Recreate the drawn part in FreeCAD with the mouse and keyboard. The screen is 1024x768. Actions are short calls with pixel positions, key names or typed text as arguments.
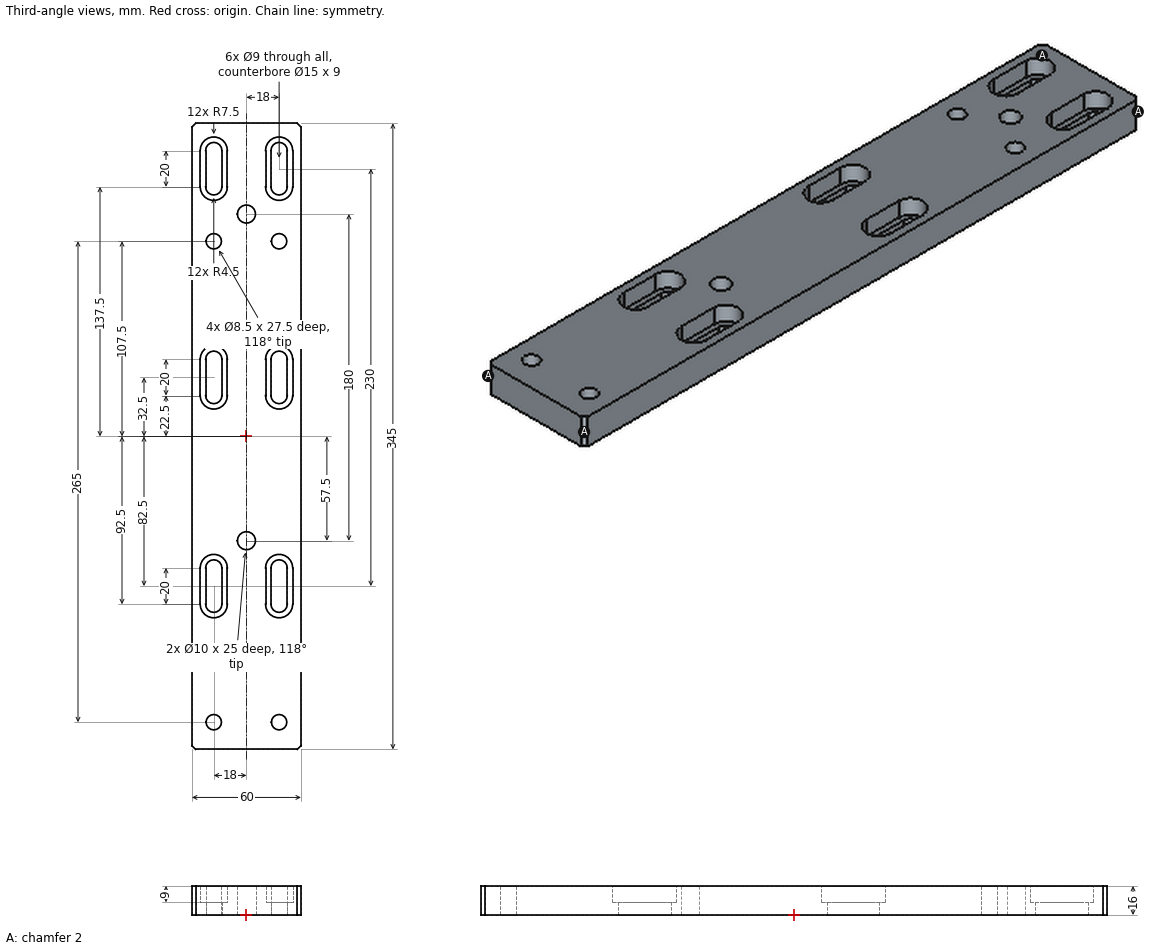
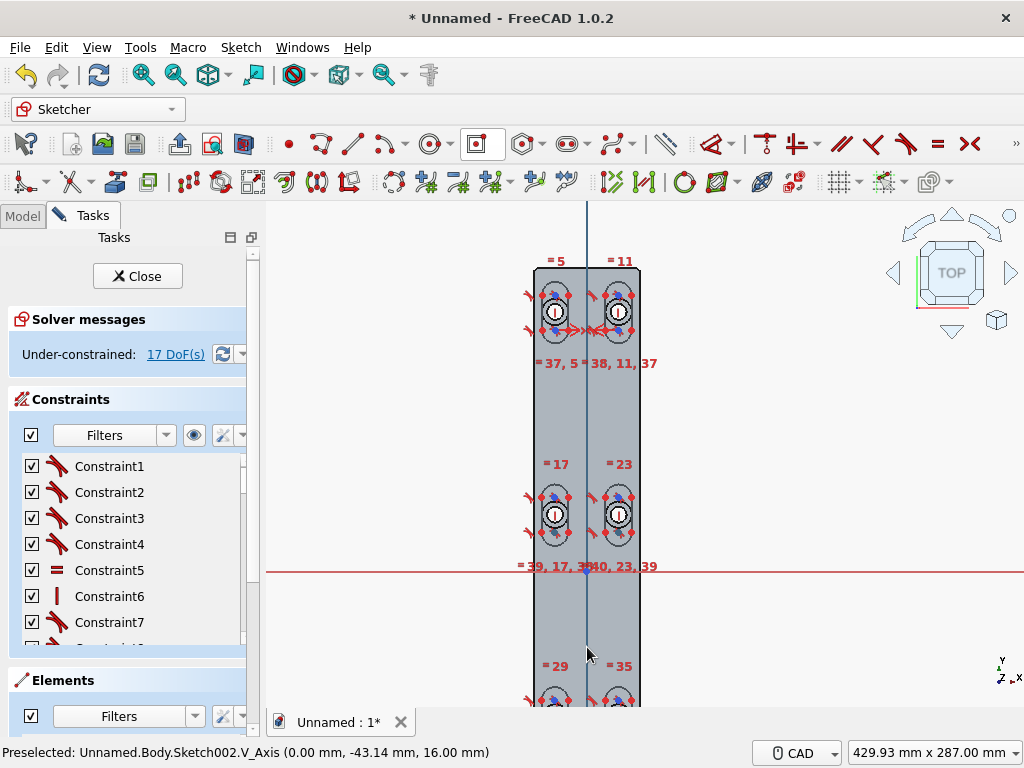
key(s)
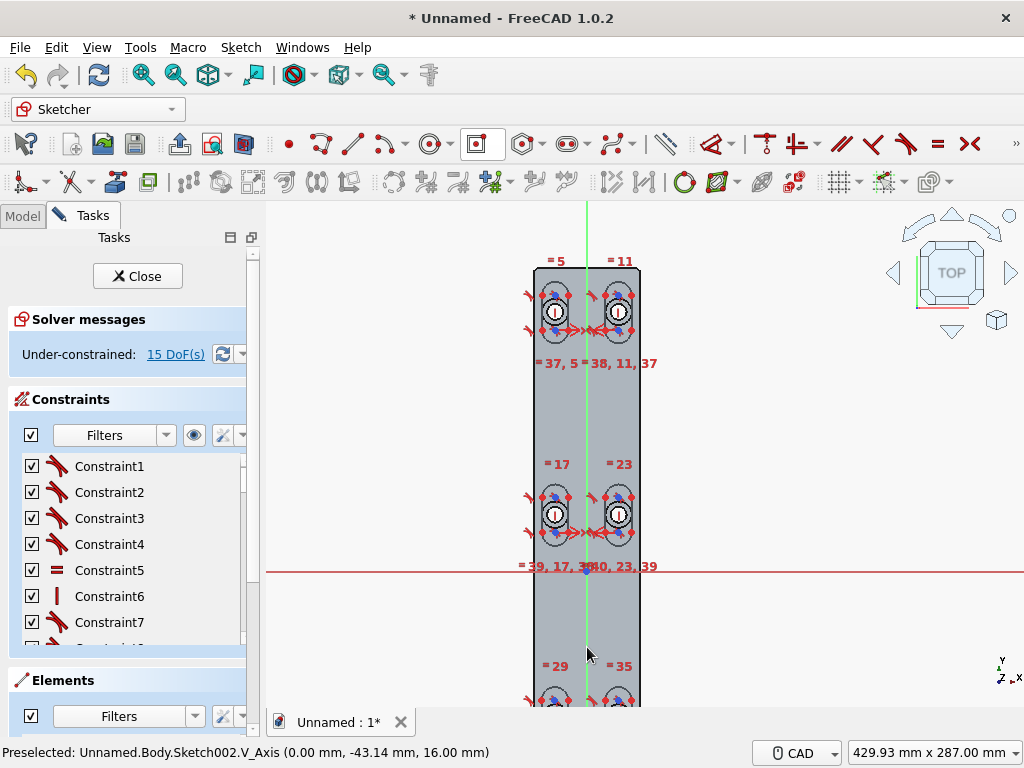
scroll(555, 331, down, 2)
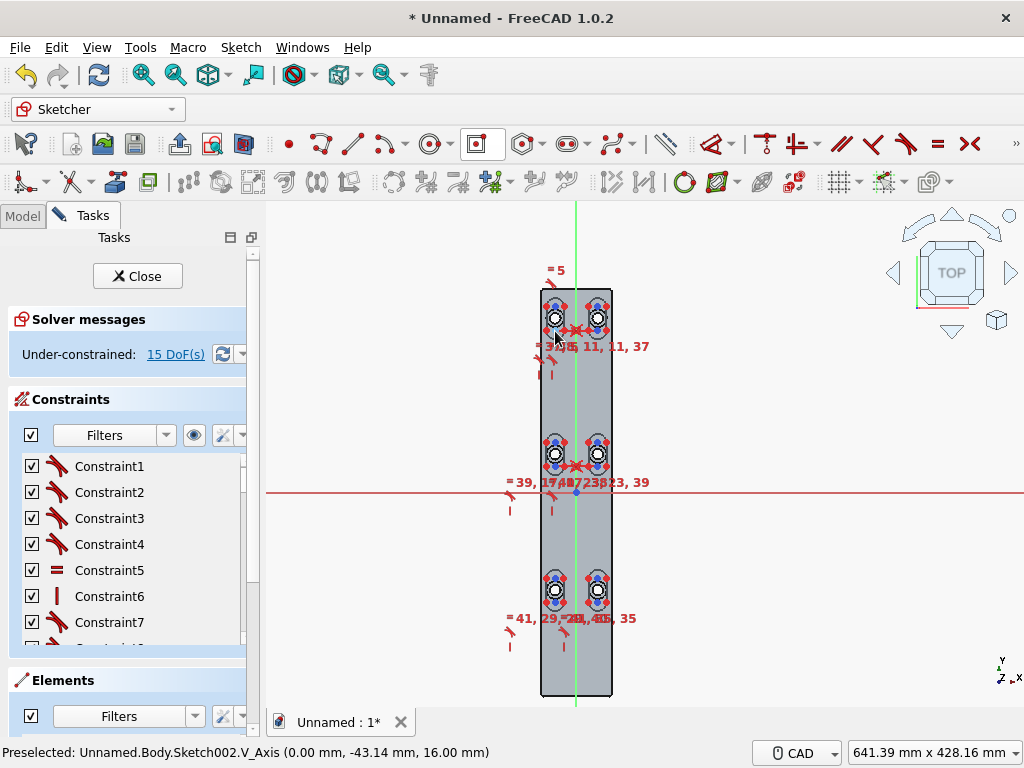
scroll(555, 602, up, 2)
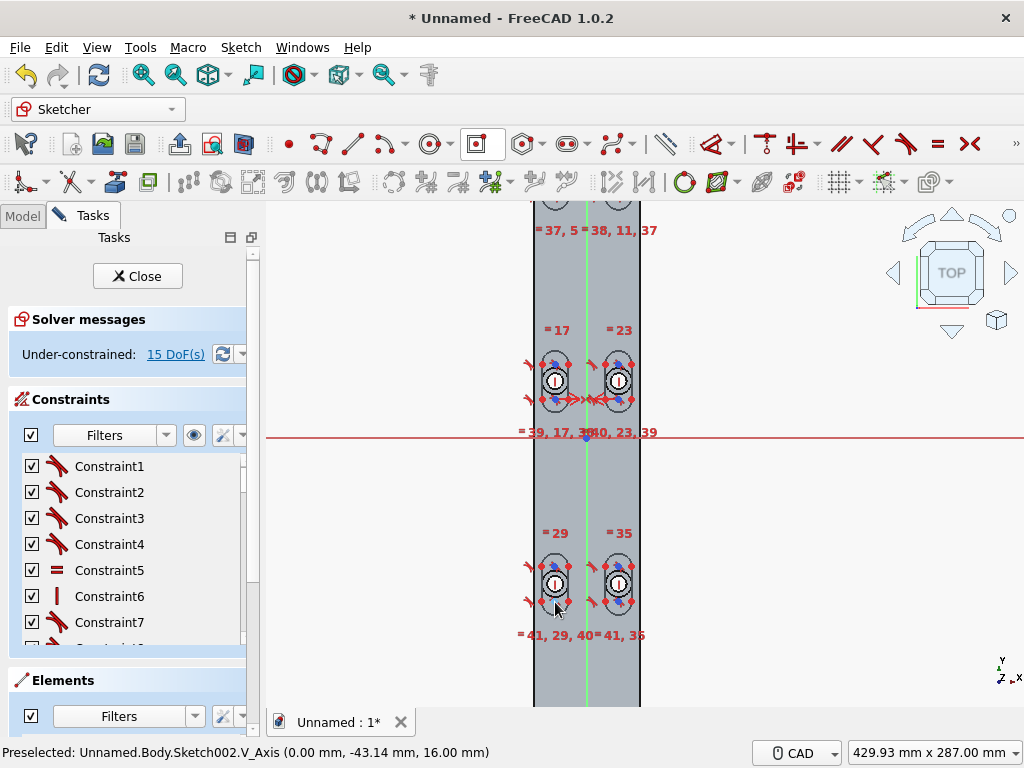
click(555, 602)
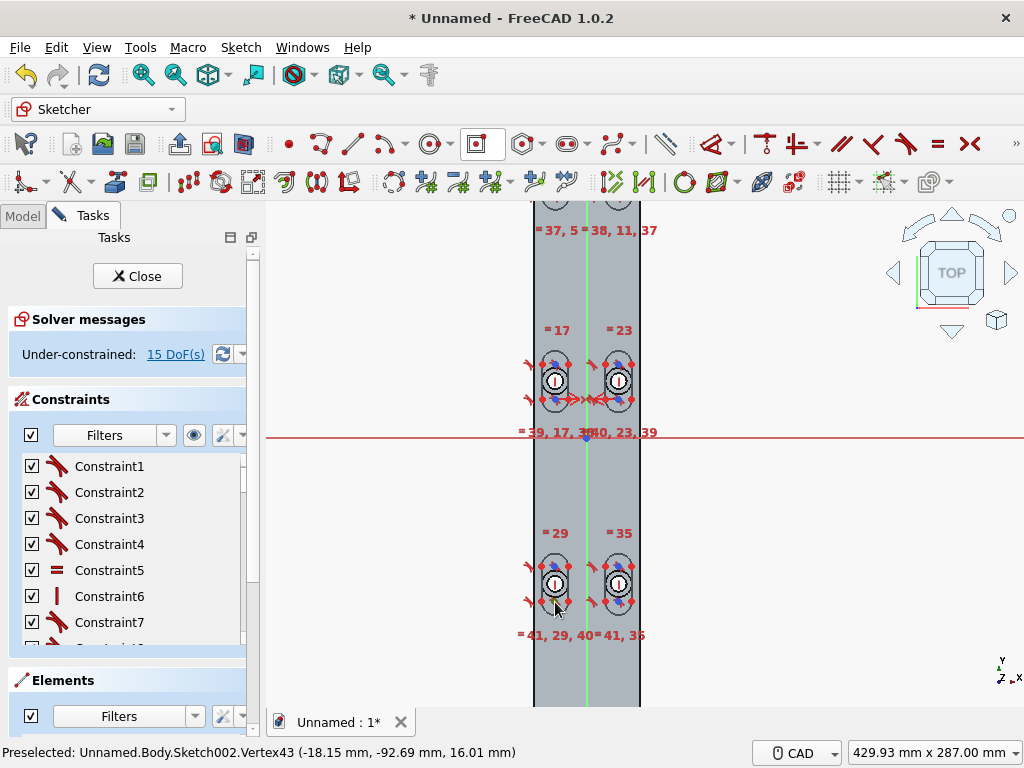
click(619, 602)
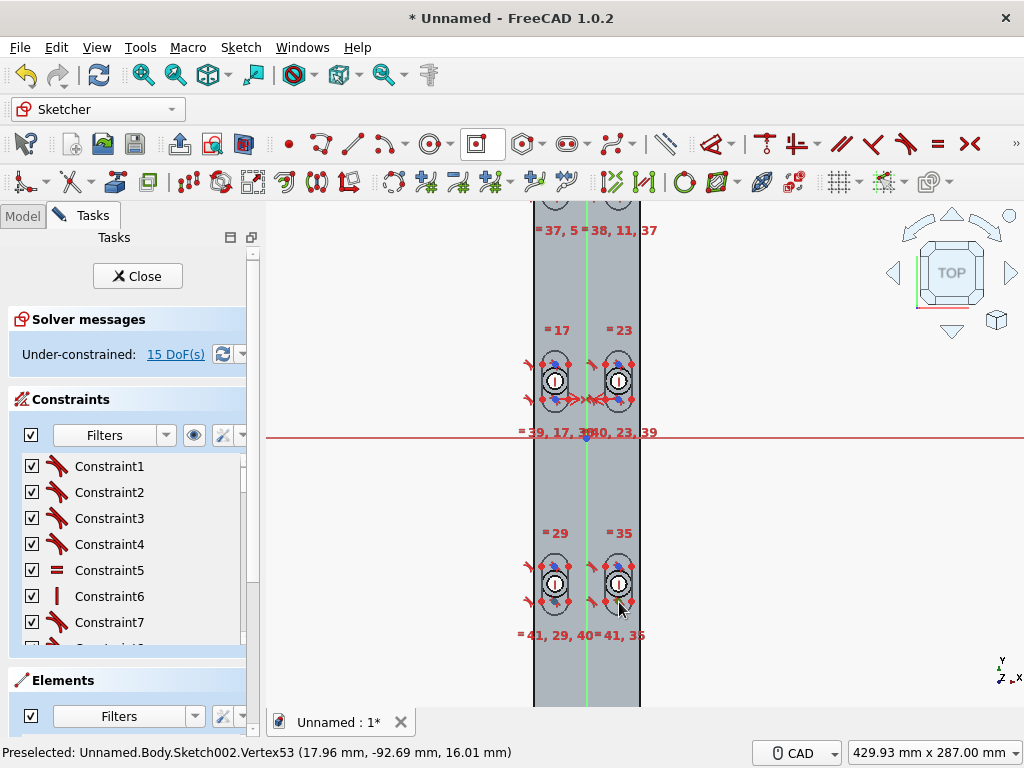
click(587, 647)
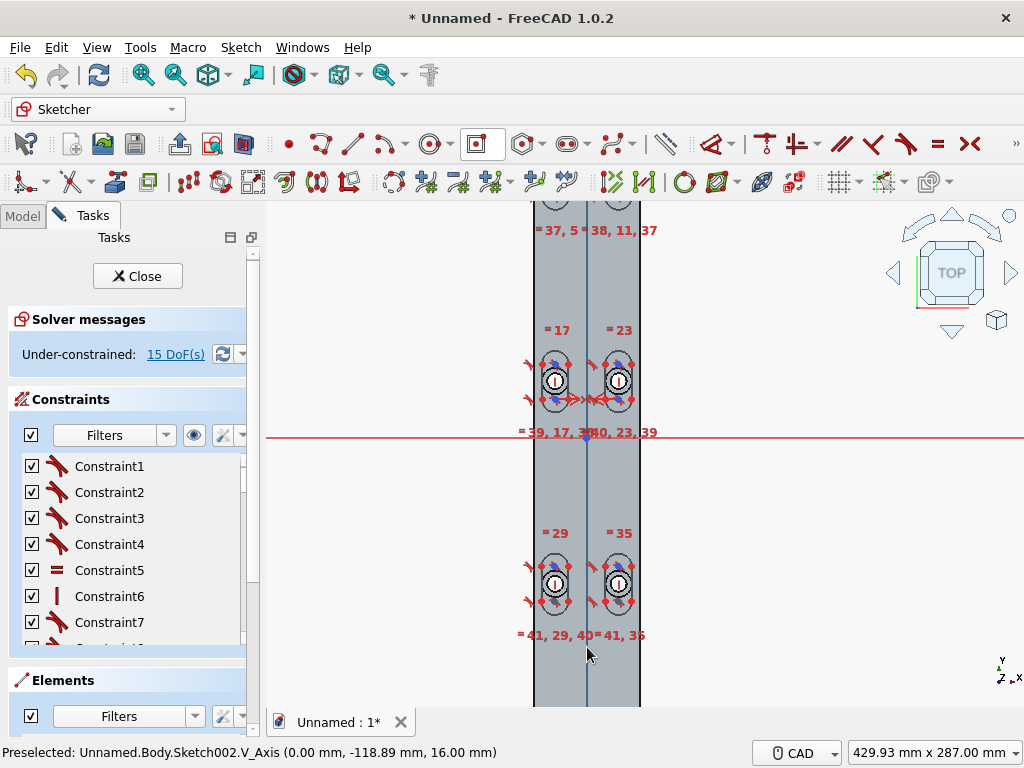
key(s)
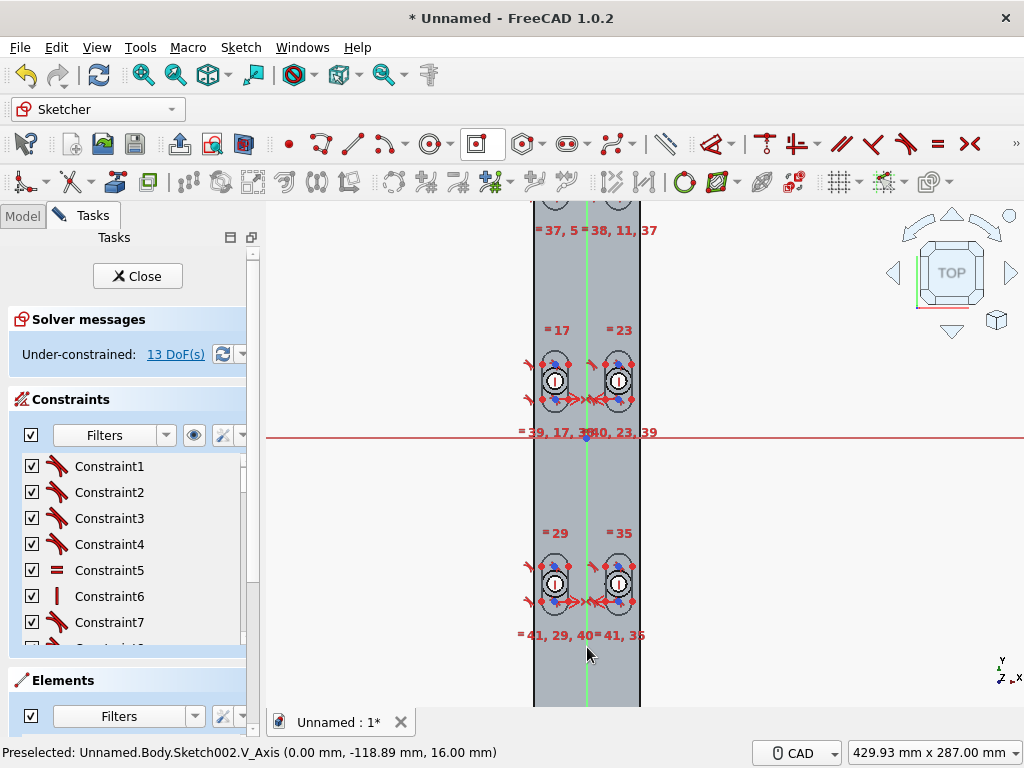
click(712, 144)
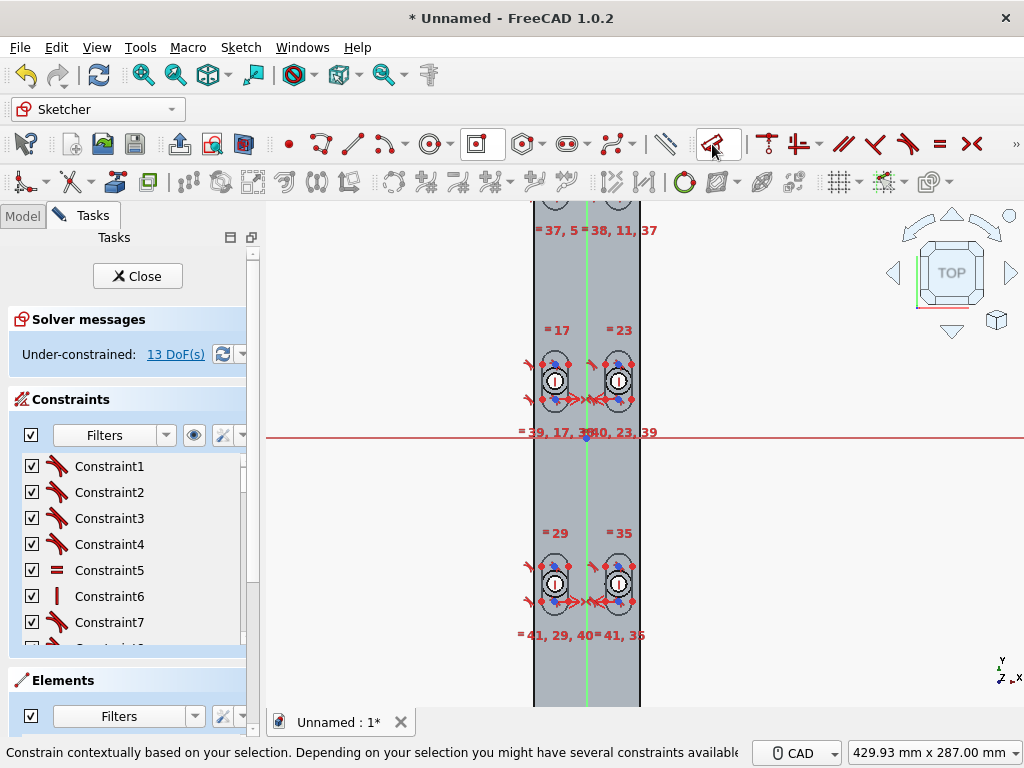
scroll(555, 602, down, 2)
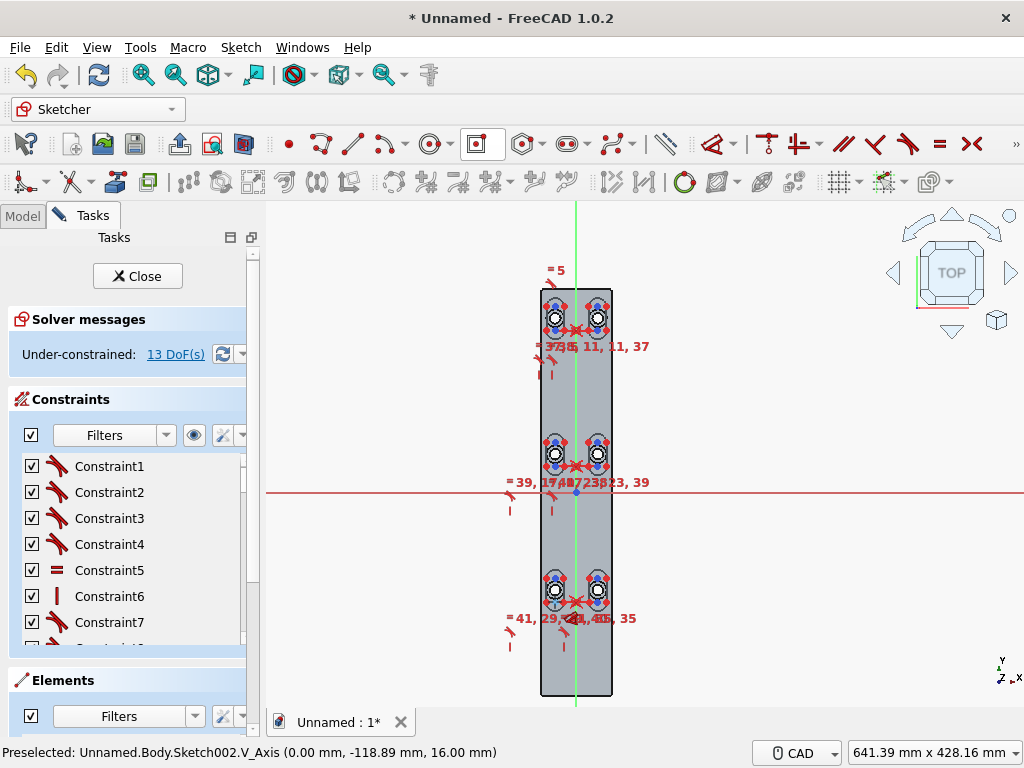
scroll(550, 338, up, 8)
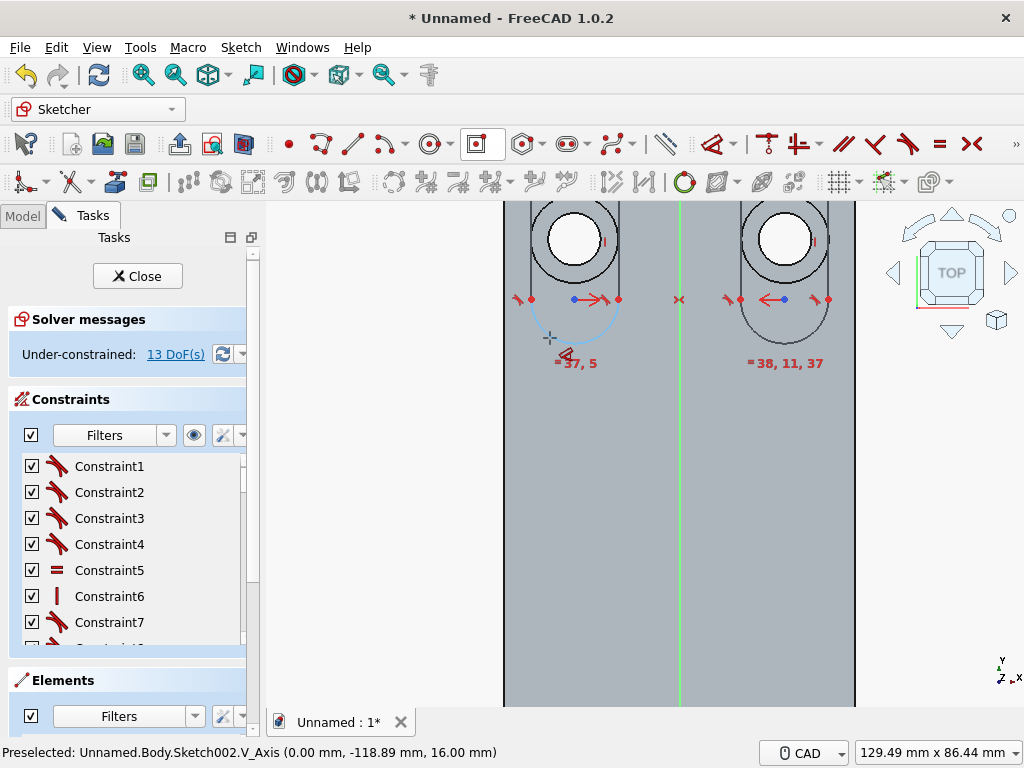
click(549, 335)
click(530, 361)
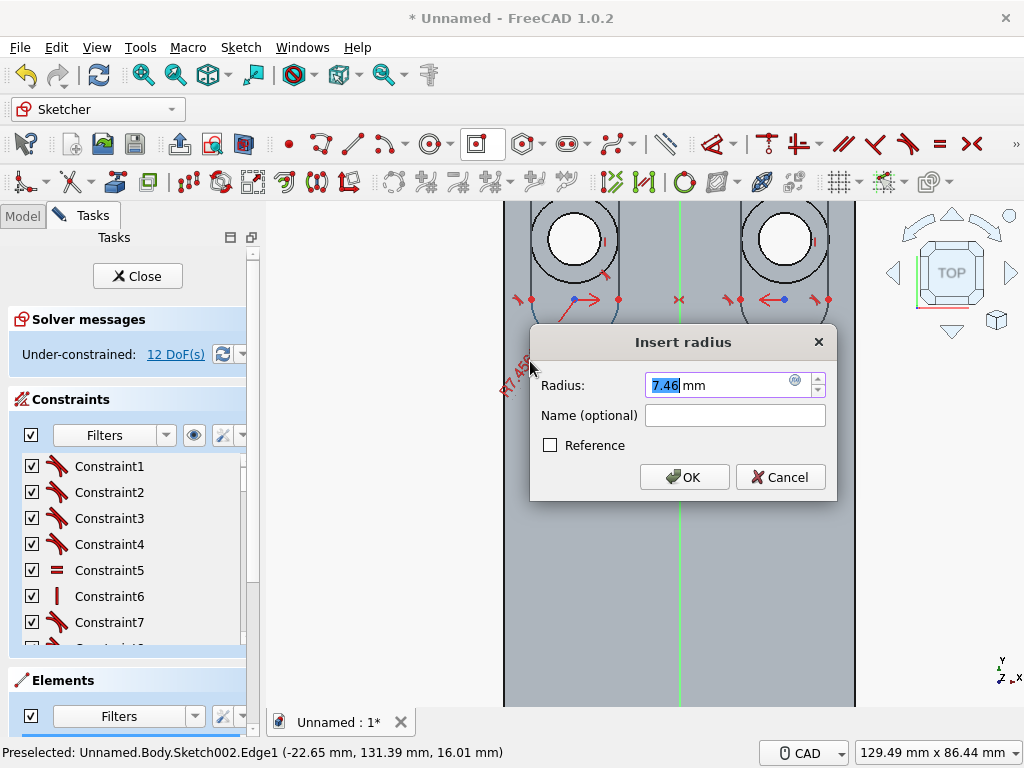
text(7.5)
key(Return)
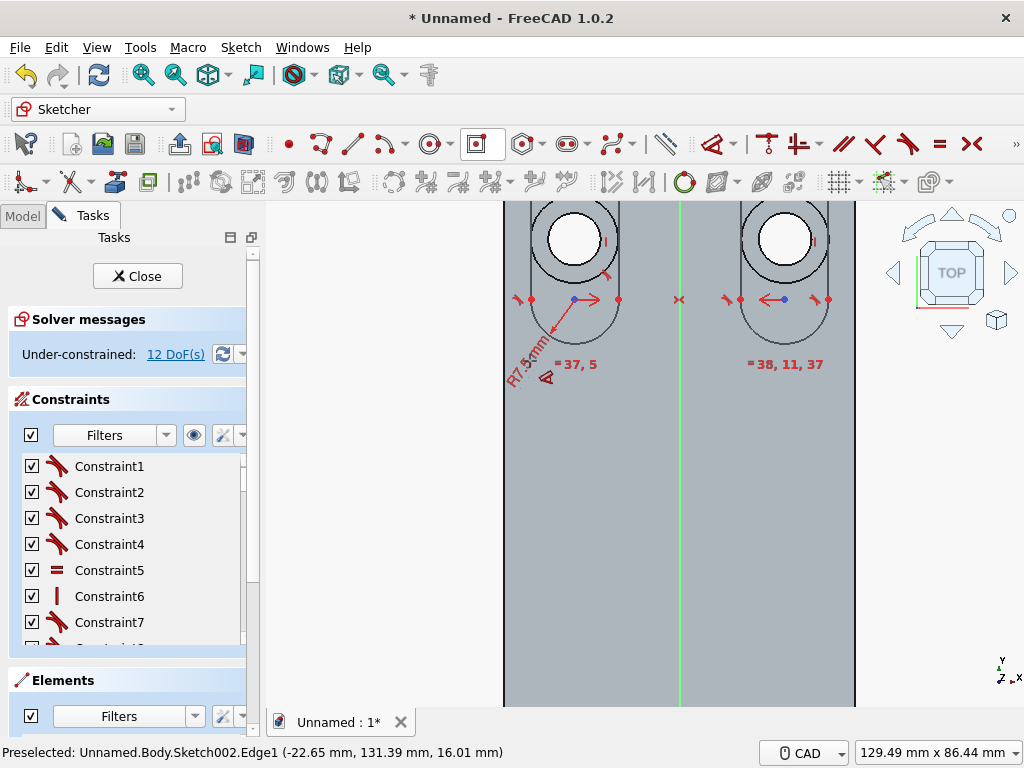
click(531, 265)
click(497, 264)